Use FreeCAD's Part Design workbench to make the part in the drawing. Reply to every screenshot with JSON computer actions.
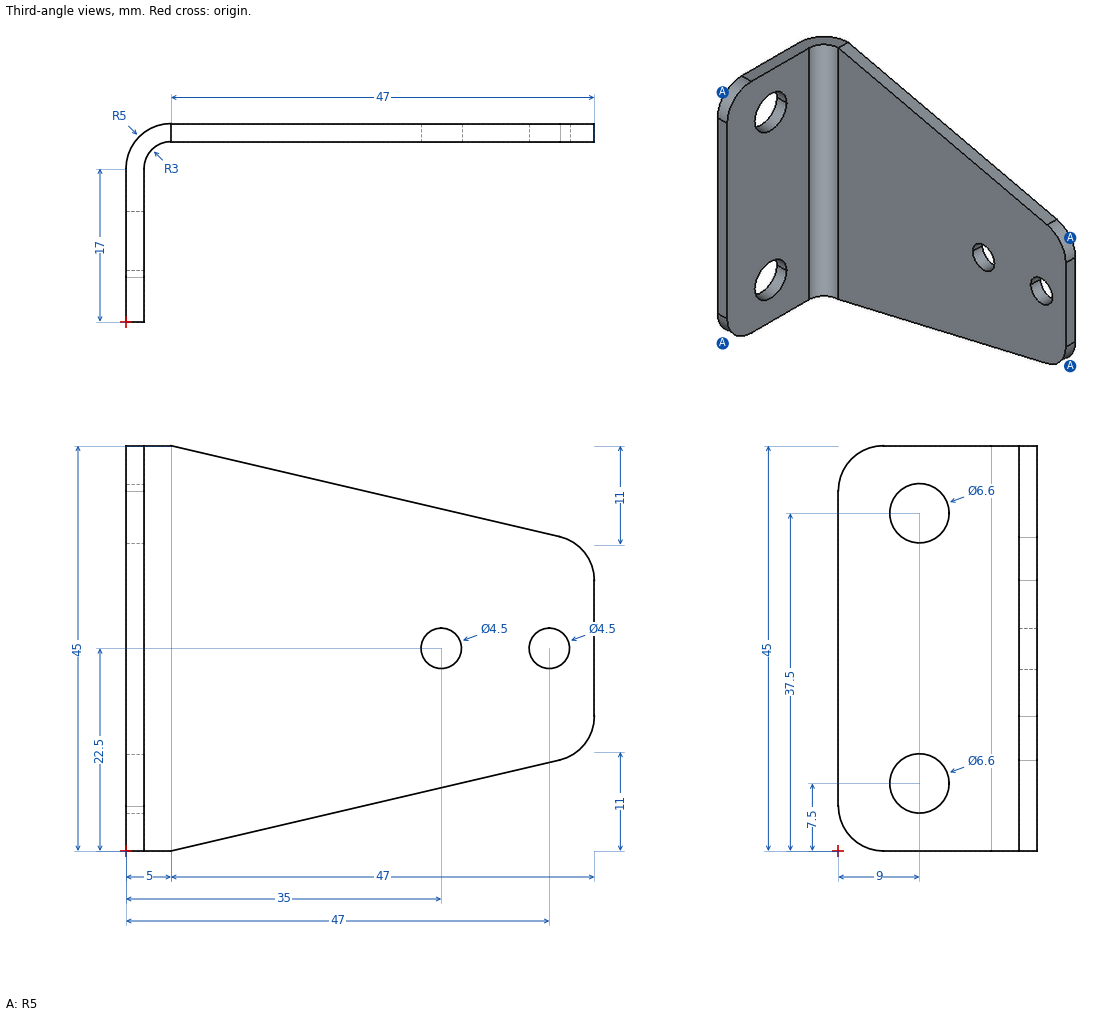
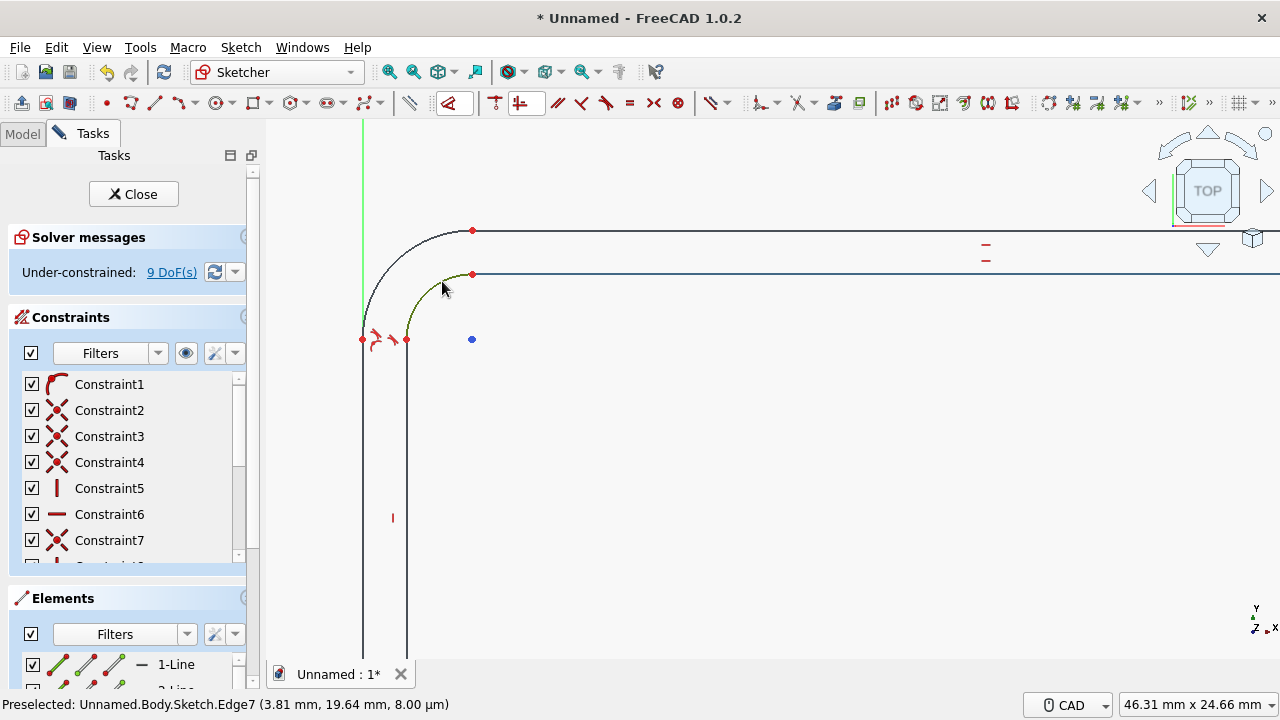
{"action": "key", "text": "t"}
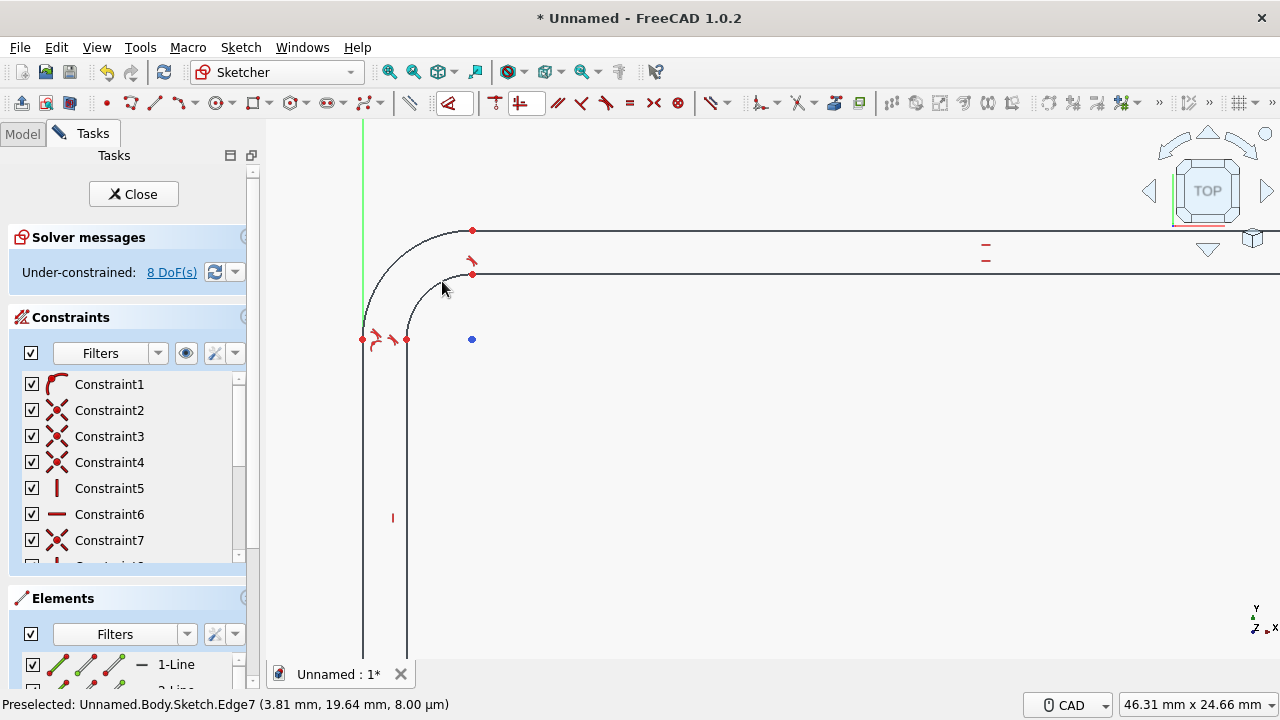
{"action": "left_click", "coordinate": [781, 231]}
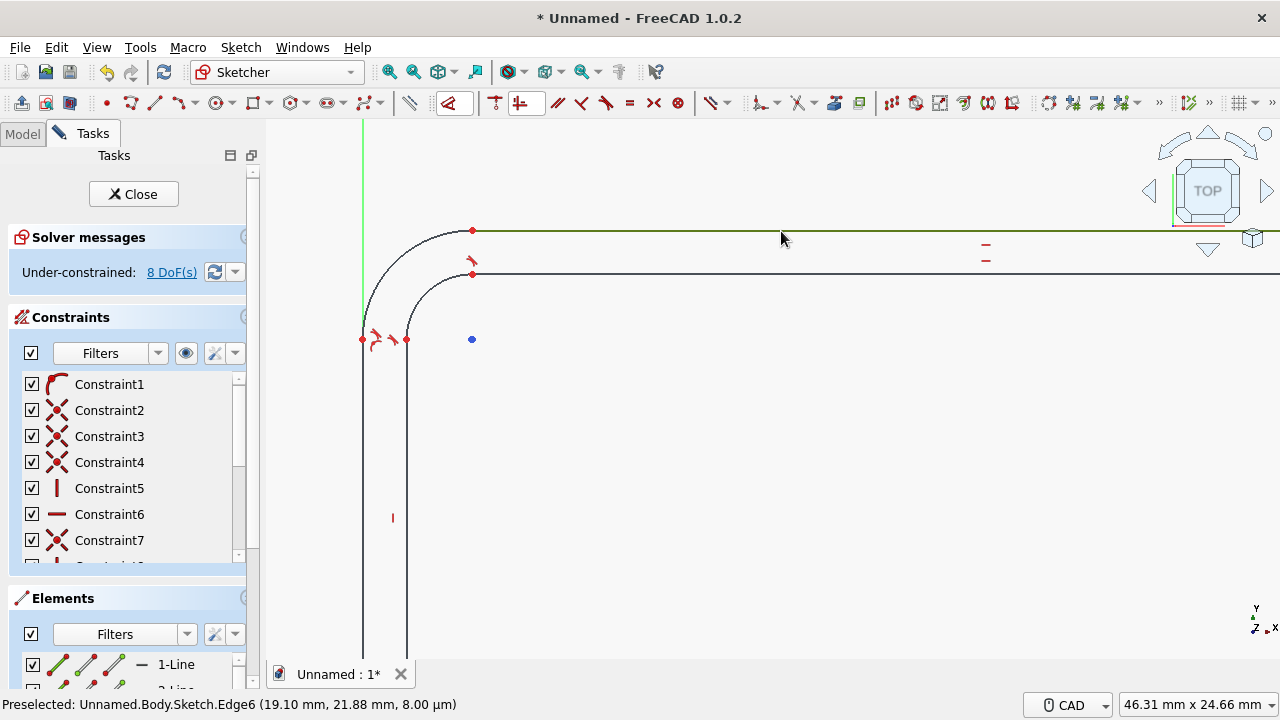
{"action": "left_click", "coordinate": [423, 242]}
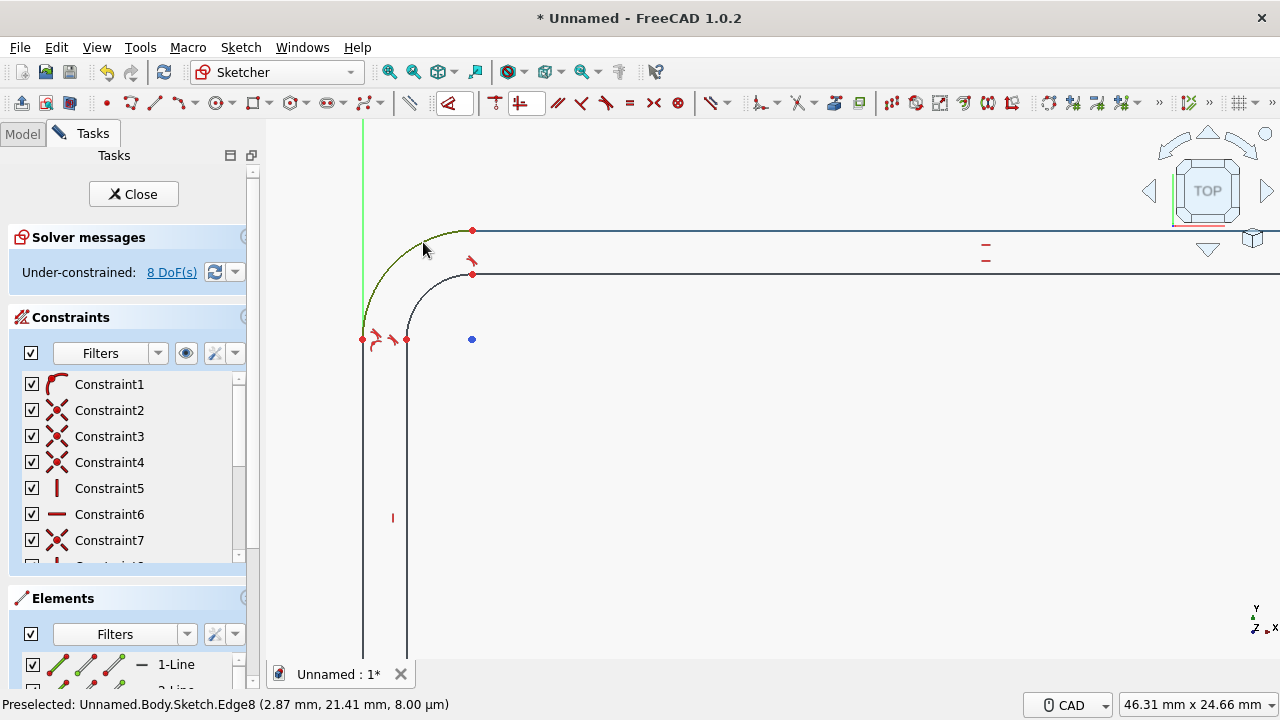
{"action": "key", "text": "t"}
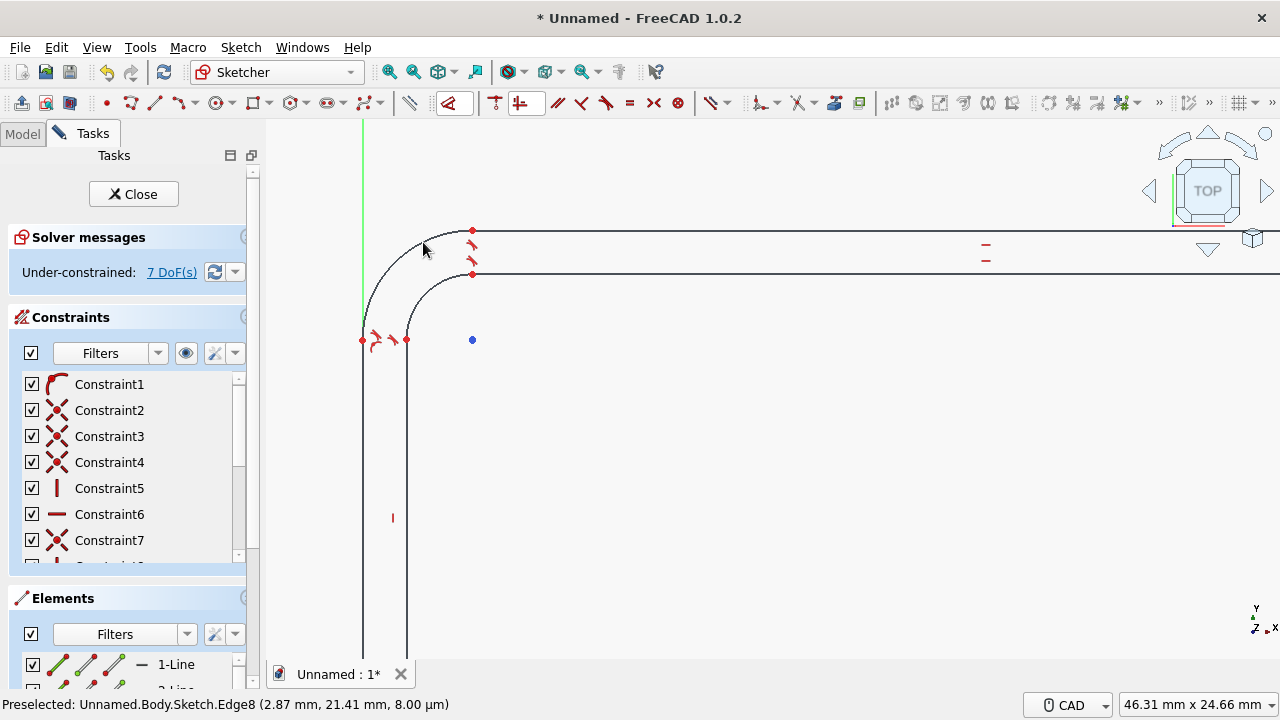
{"action": "scroll", "coordinate": [428, 292], "scroll_direction": "down", "scroll_amount": 3}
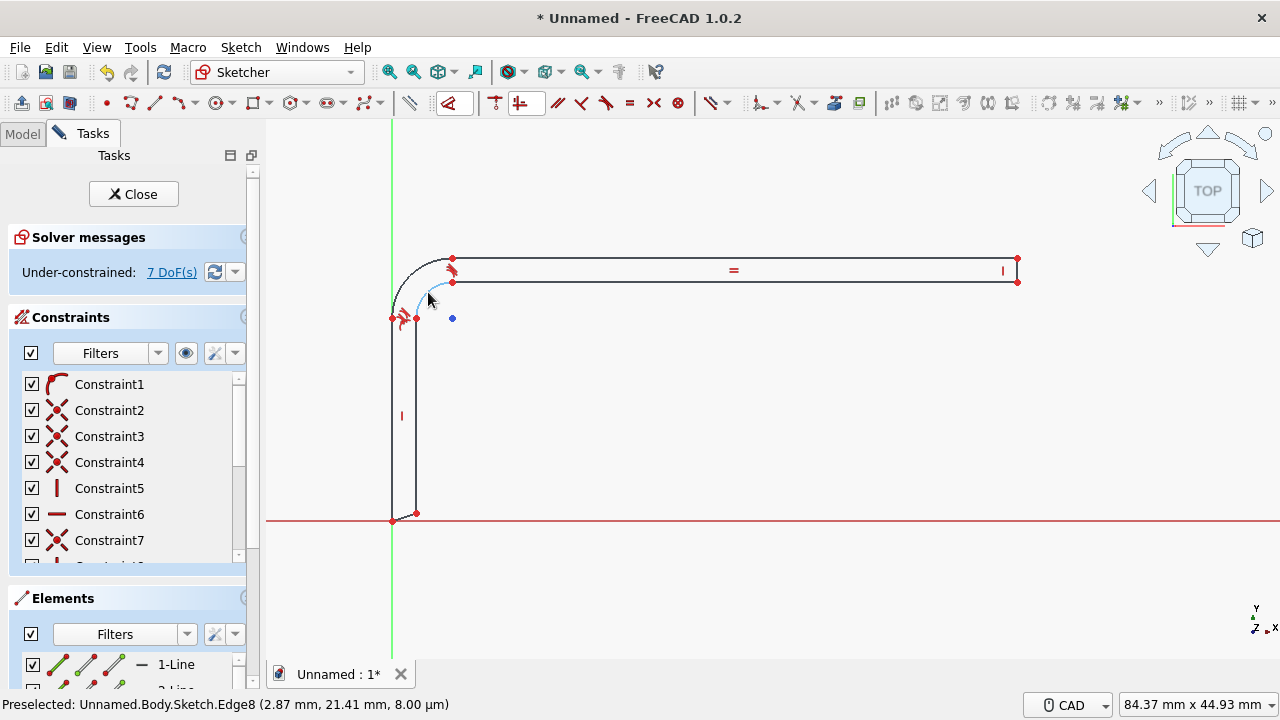
{"action": "scroll", "coordinate": [409, 516], "scroll_direction": "up", "scroll_amount": 5}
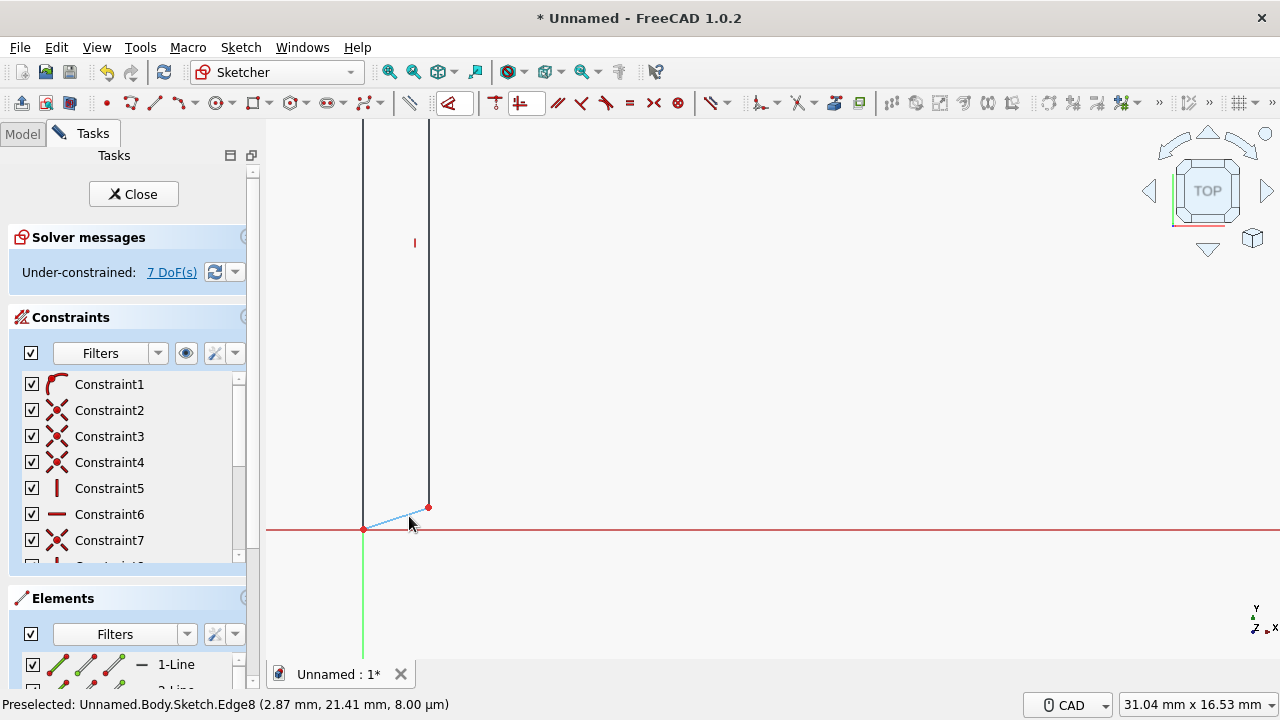
{"action": "left_click", "coordinate": [409, 514]}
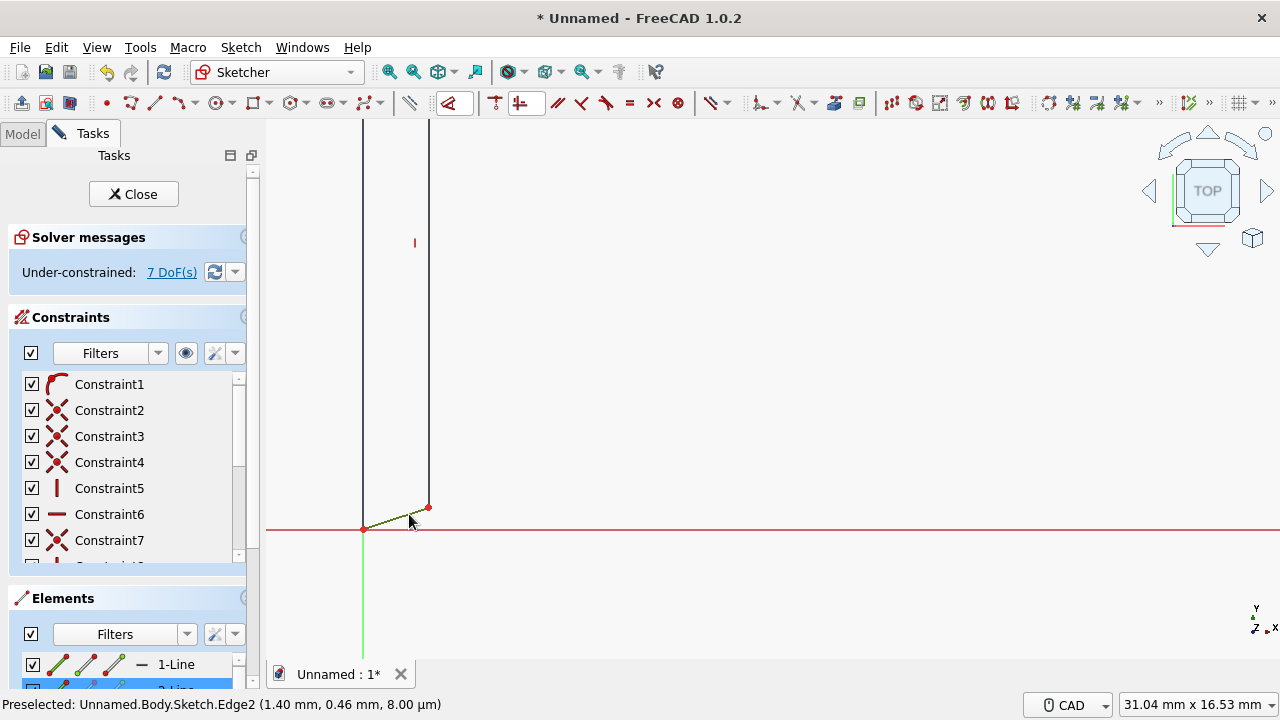
{"action": "key", "text": "h"}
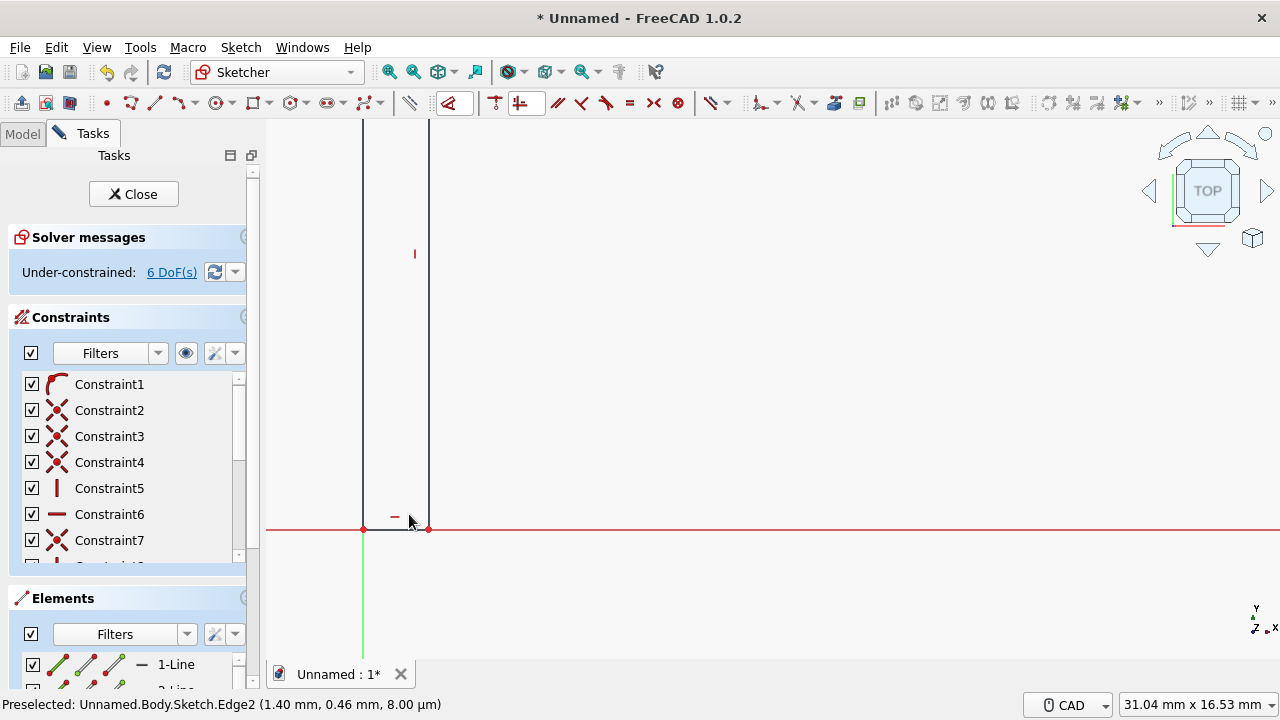
{"action": "scroll", "coordinate": [409, 516], "scroll_direction": "down", "scroll_amount": 5}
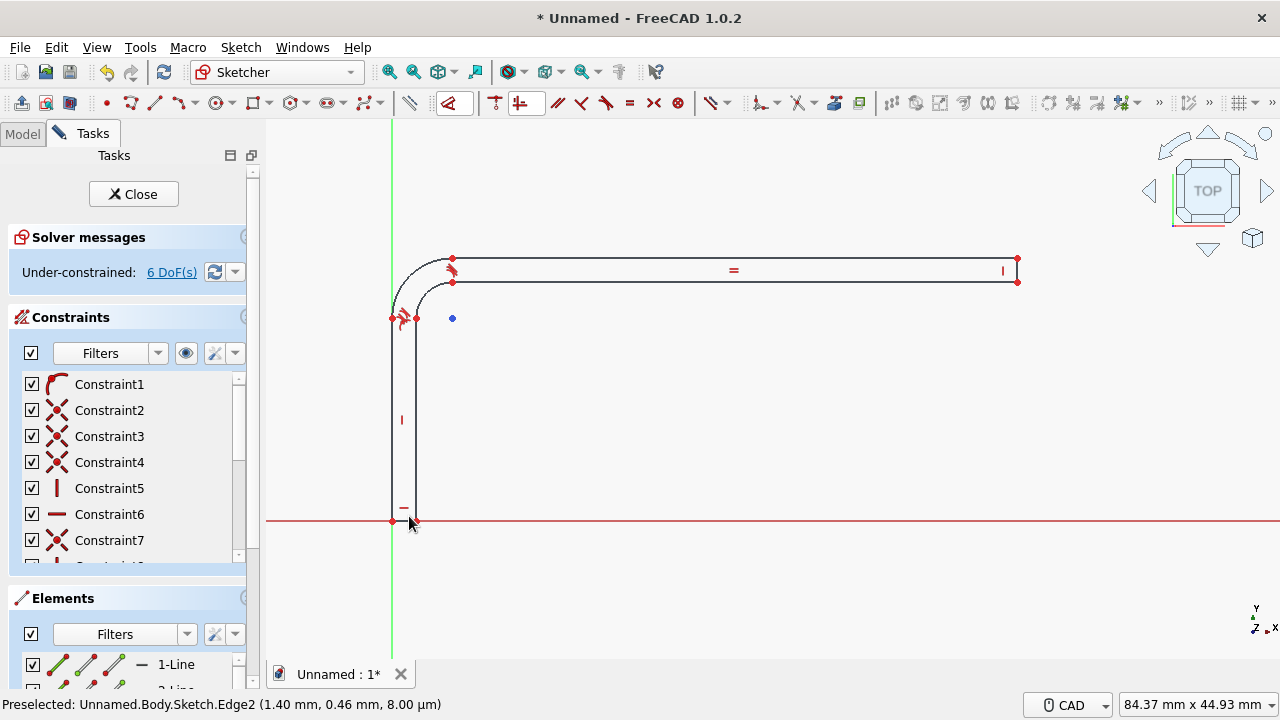
{"action": "left_click", "coordinate": [436, 286]}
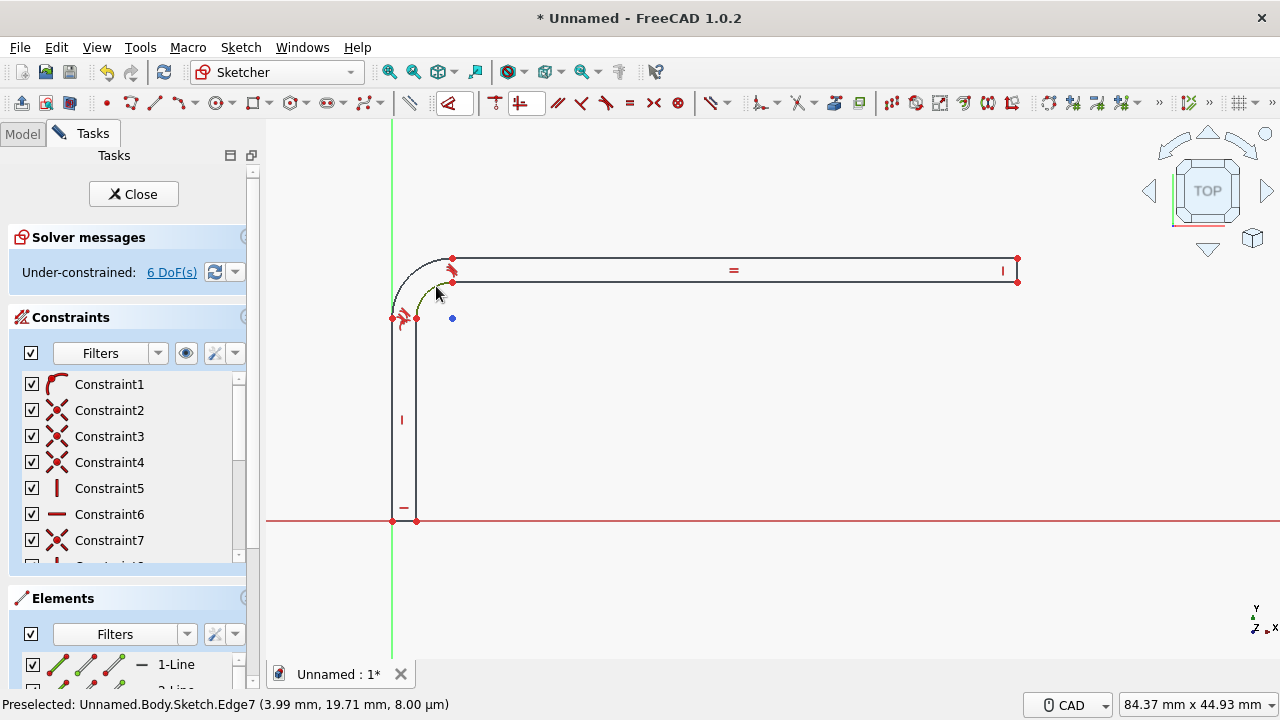
{"action": "left_click", "coordinate": [425, 265]}